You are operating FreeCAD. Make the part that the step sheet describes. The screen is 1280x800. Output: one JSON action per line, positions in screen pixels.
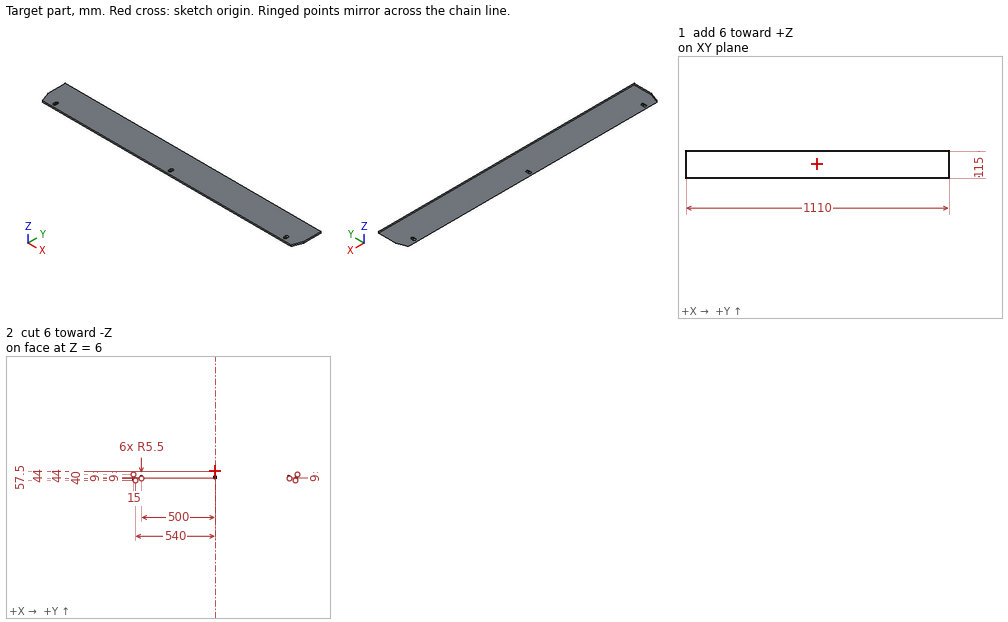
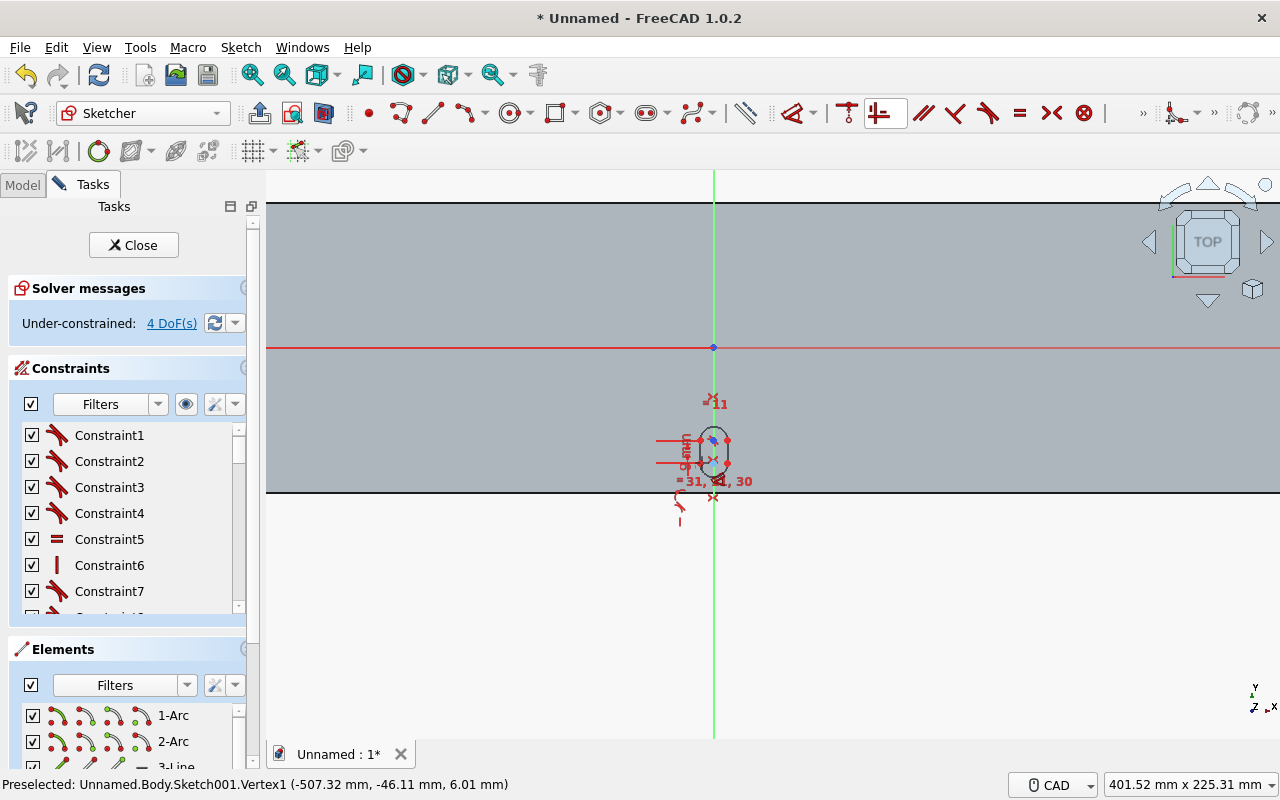
{"action": "left_click", "coordinate": [700, 463]}
{"action": "left_click", "coordinate": [666, 406]}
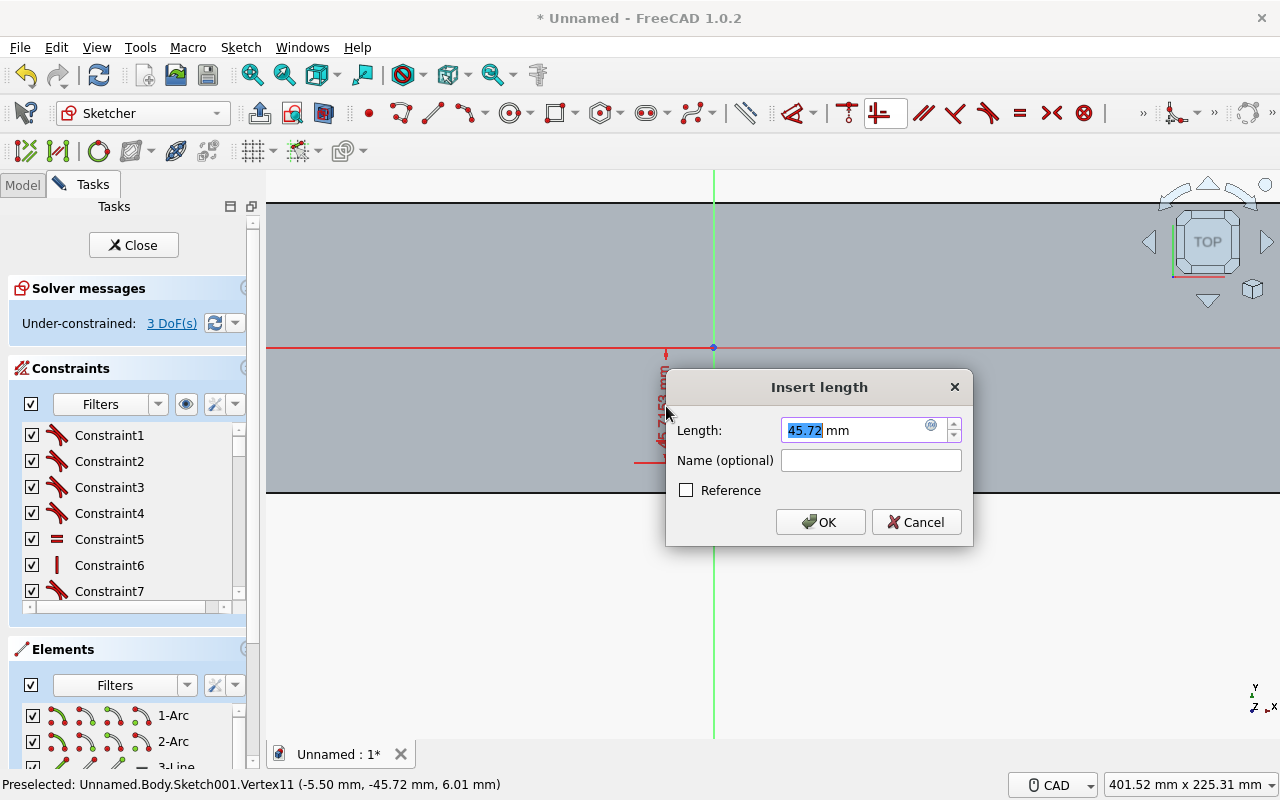
{"action": "type", "text": "44"}
{"action": "key", "text": "Return"}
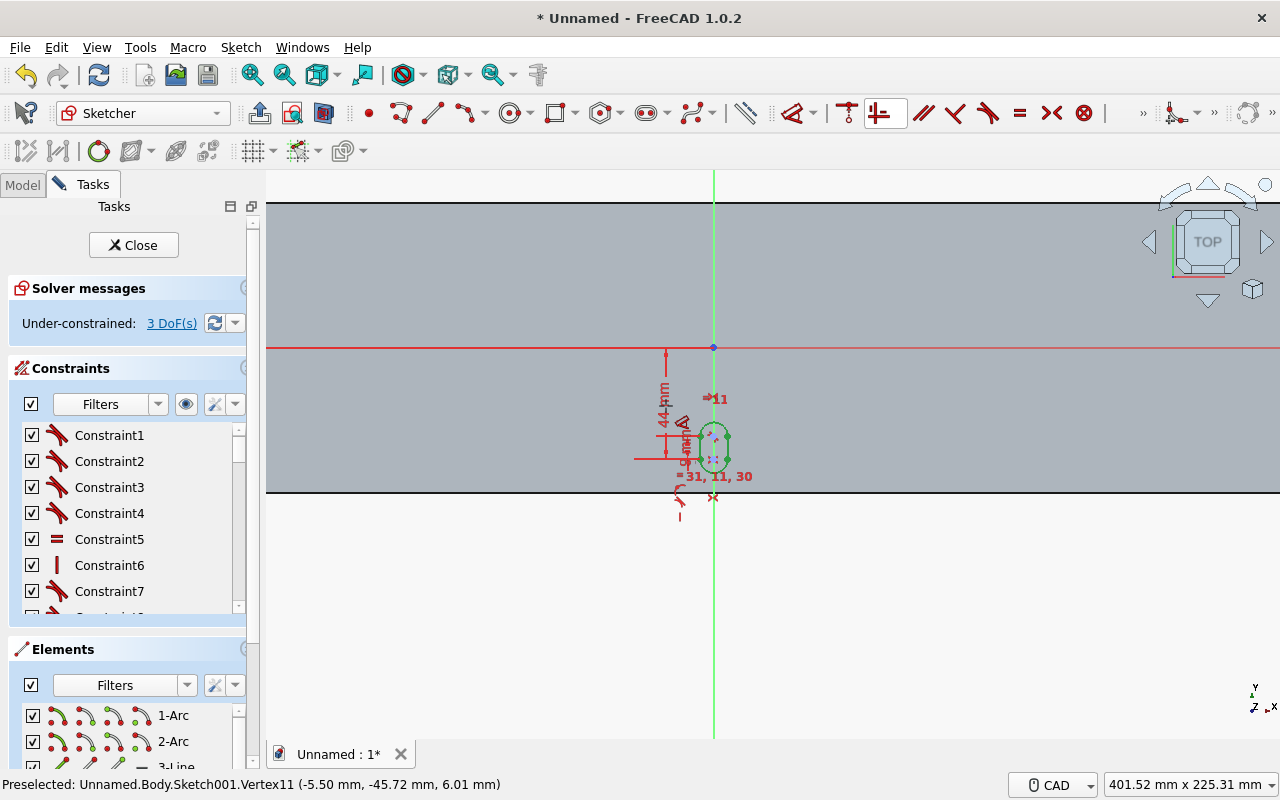
{"action": "scroll", "coordinate": [702, 463], "scroll_direction": "down", "scroll_amount": 8}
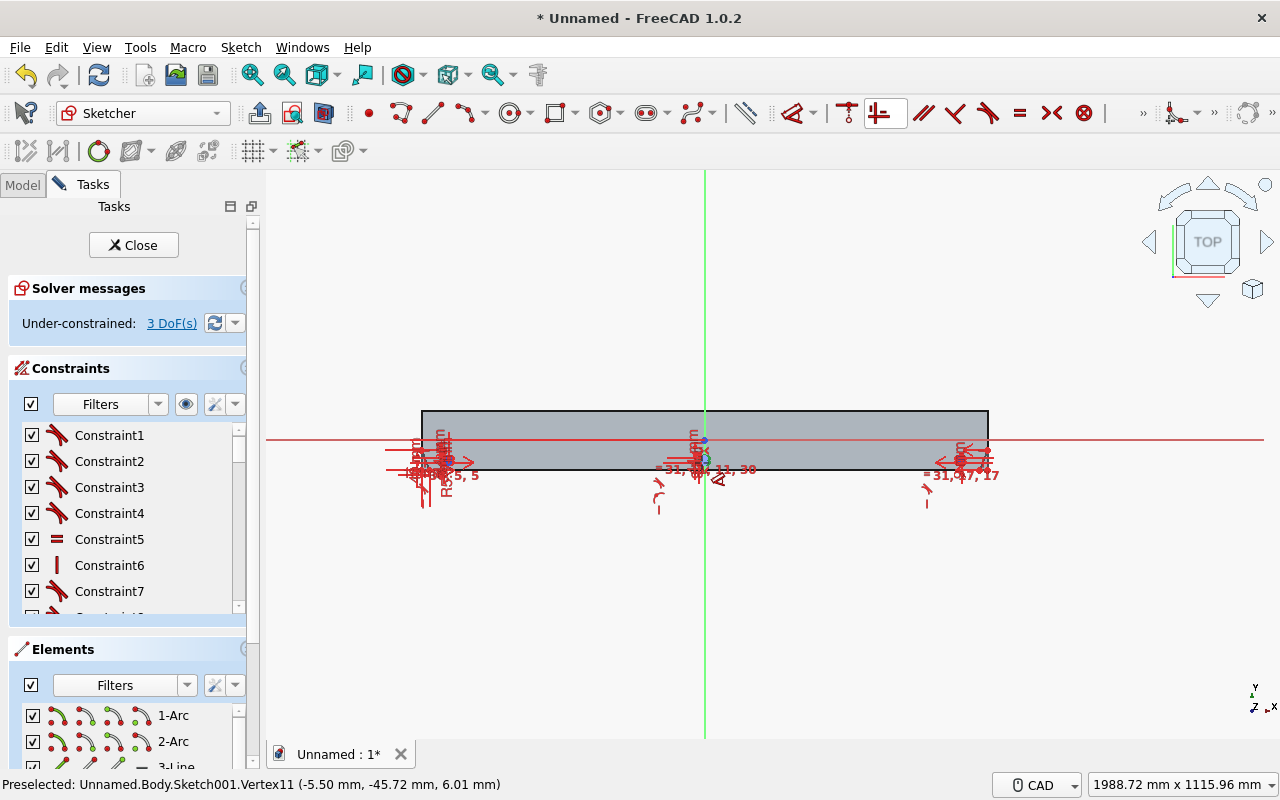
{"action": "scroll", "coordinate": [430, 470], "scroll_direction": "up", "scroll_amount": 3}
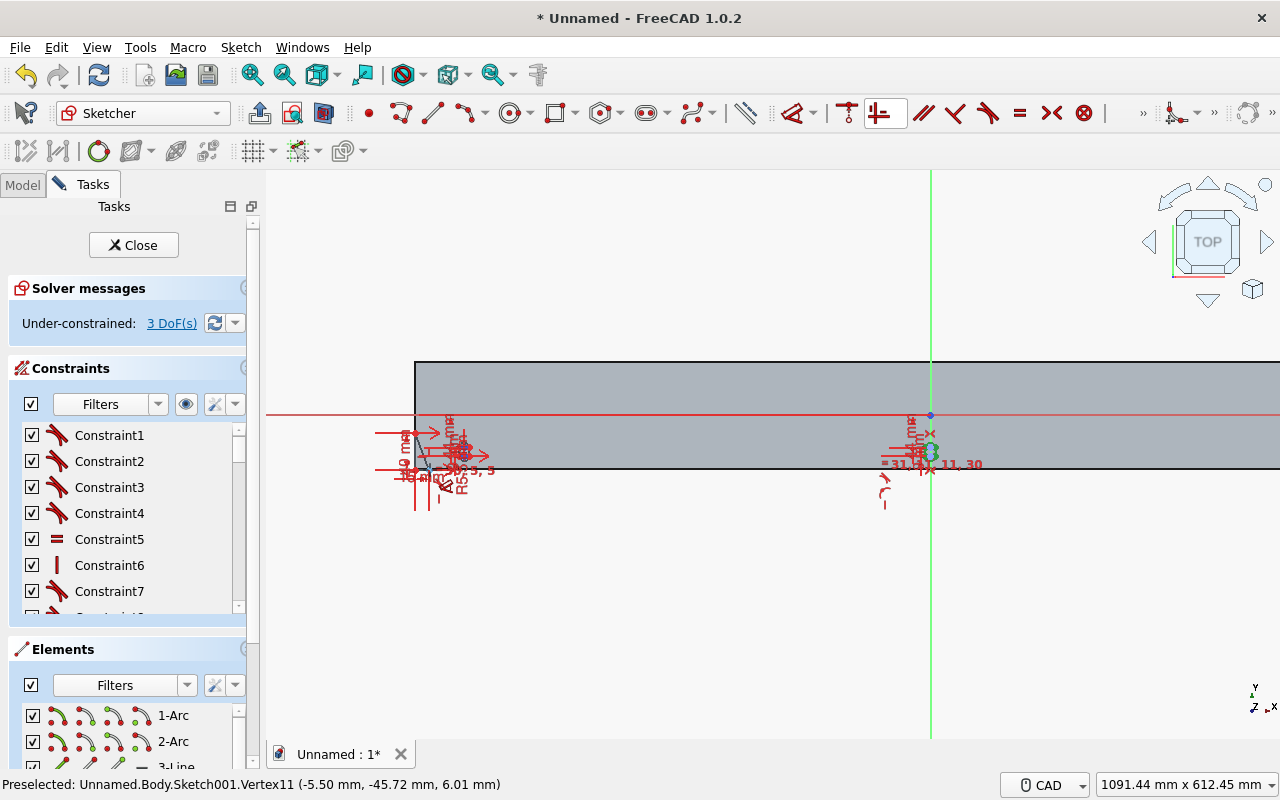
{"action": "left_click", "coordinate": [429, 470]}
{"action": "left_click", "coordinate": [680, 504]}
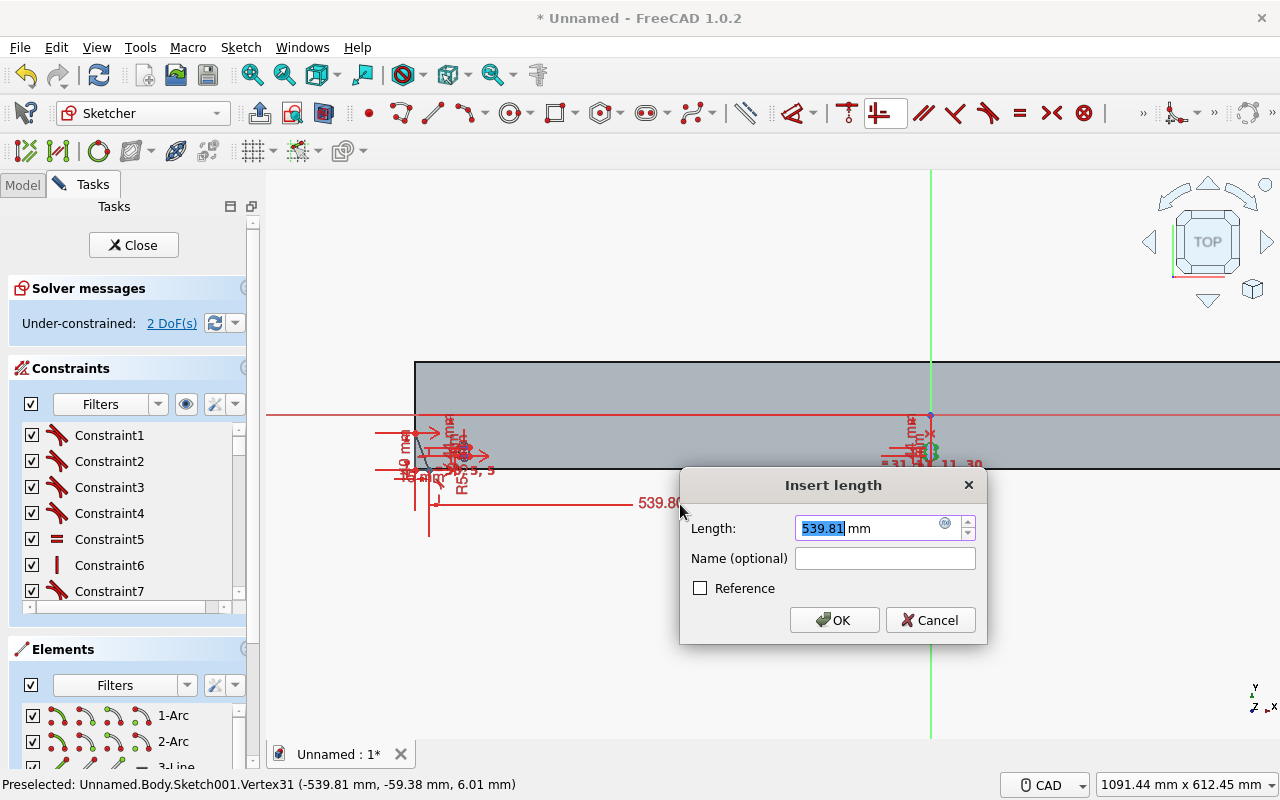
{"action": "type", "text": "540"}
{"action": "key", "text": "Return"}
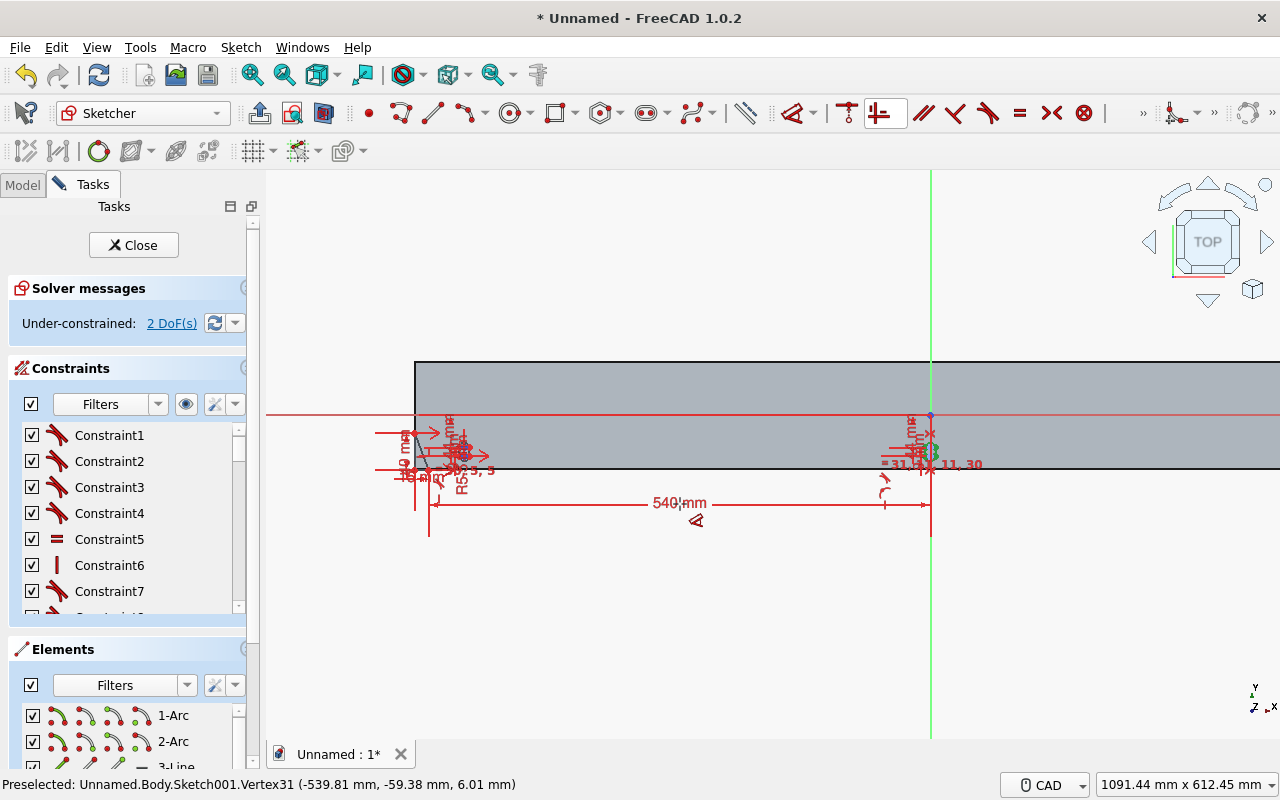
{"action": "scroll", "coordinate": [464, 456], "scroll_direction": "up", "scroll_amount": 5}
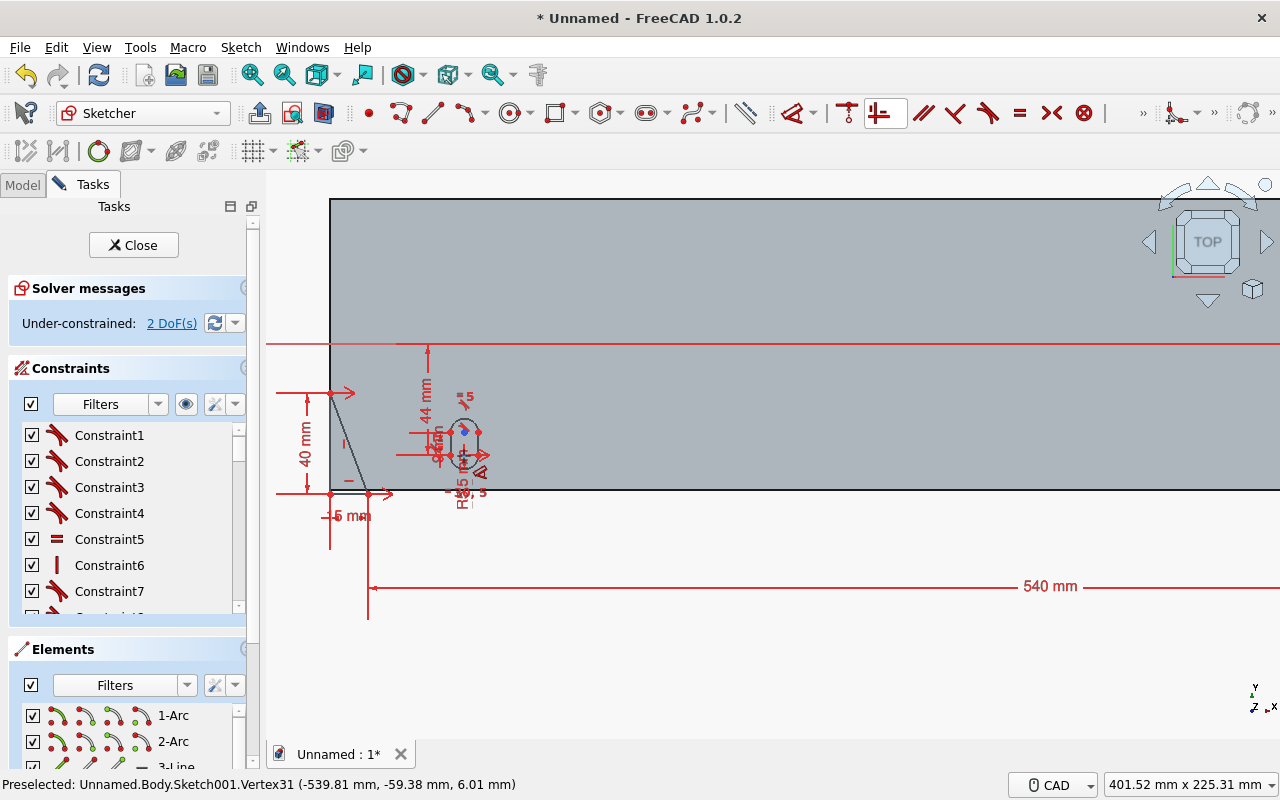
{"action": "left_click", "coordinate": [464, 455]}
{"action": "left_click", "coordinate": [790, 310]}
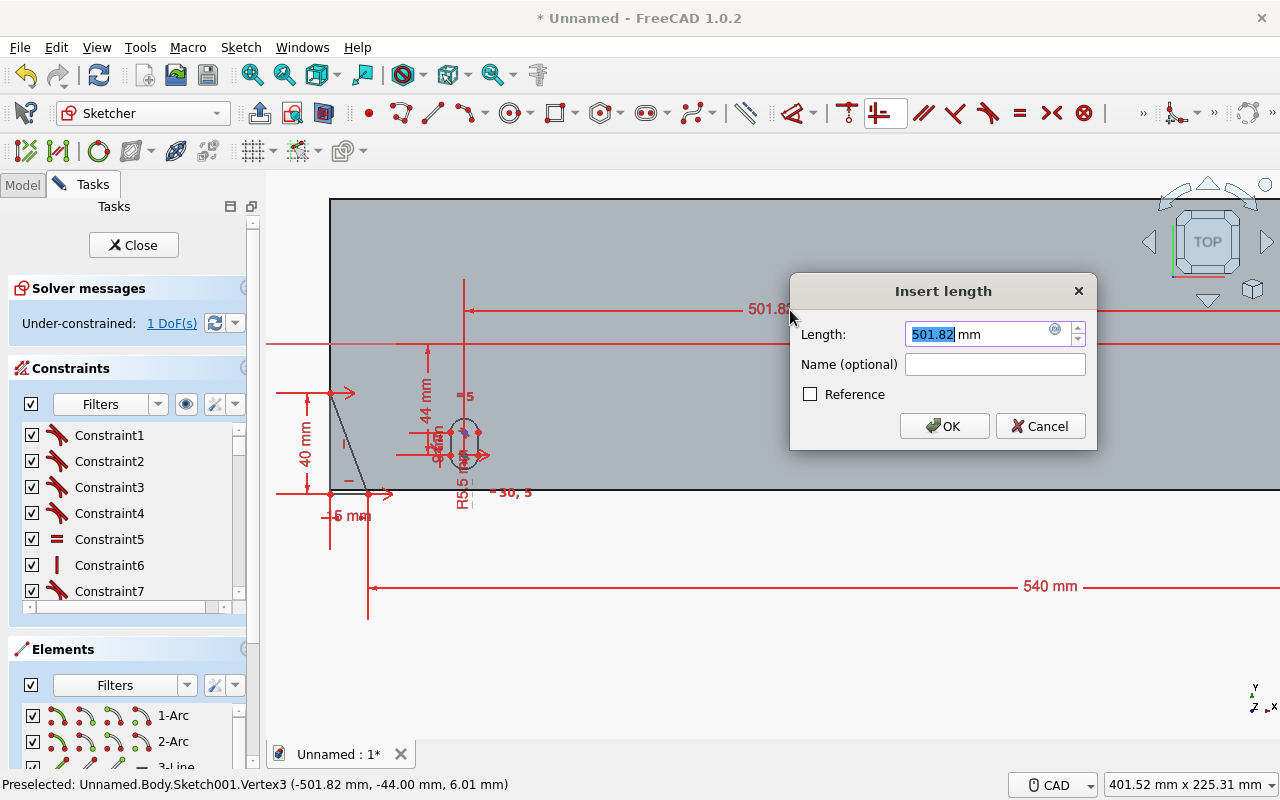
{"action": "type", "text": "500"}
{"action": "key", "text": "Return"}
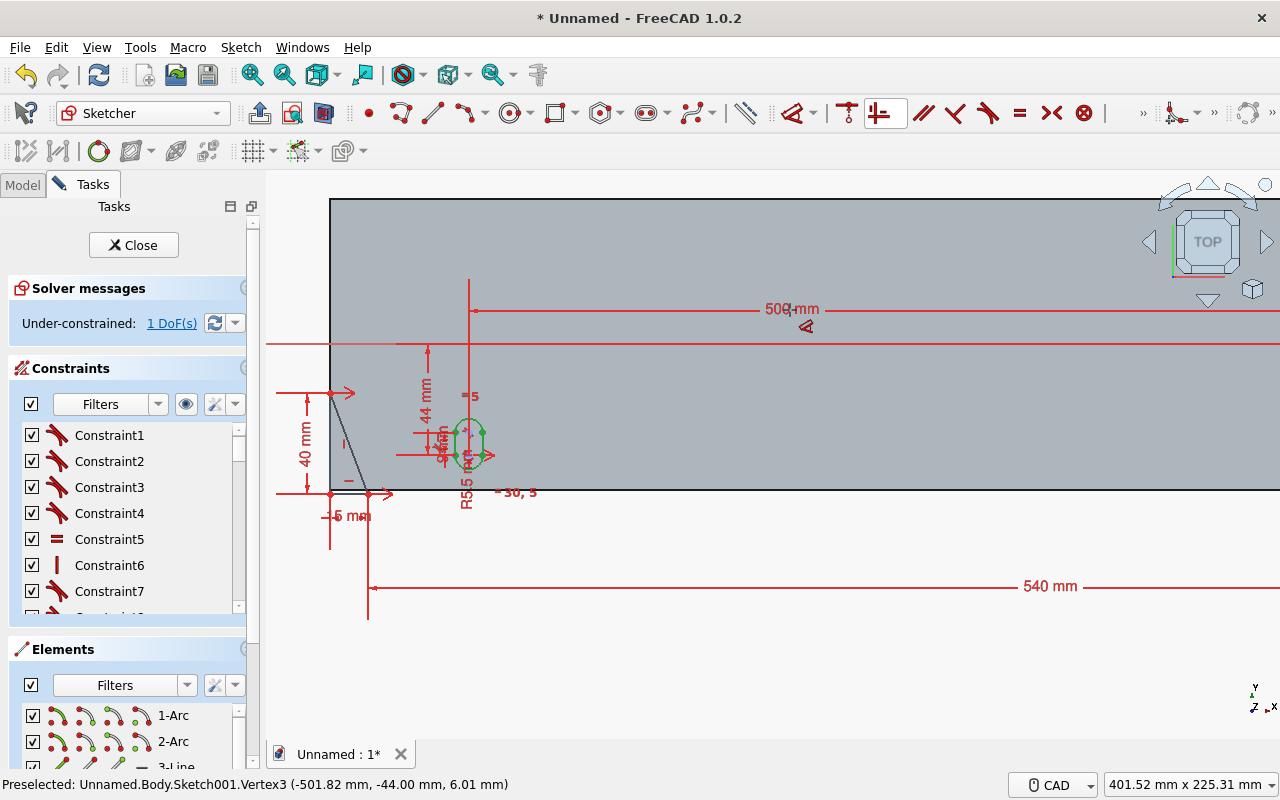
{"action": "scroll", "coordinate": [445, 464], "scroll_direction": "down", "scroll_amount": 8}